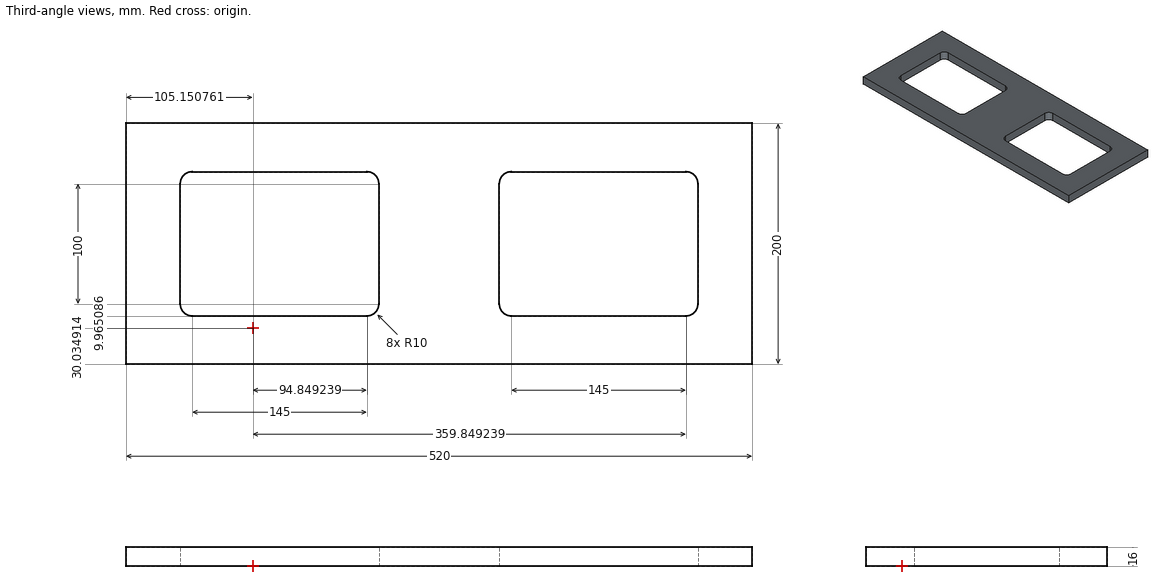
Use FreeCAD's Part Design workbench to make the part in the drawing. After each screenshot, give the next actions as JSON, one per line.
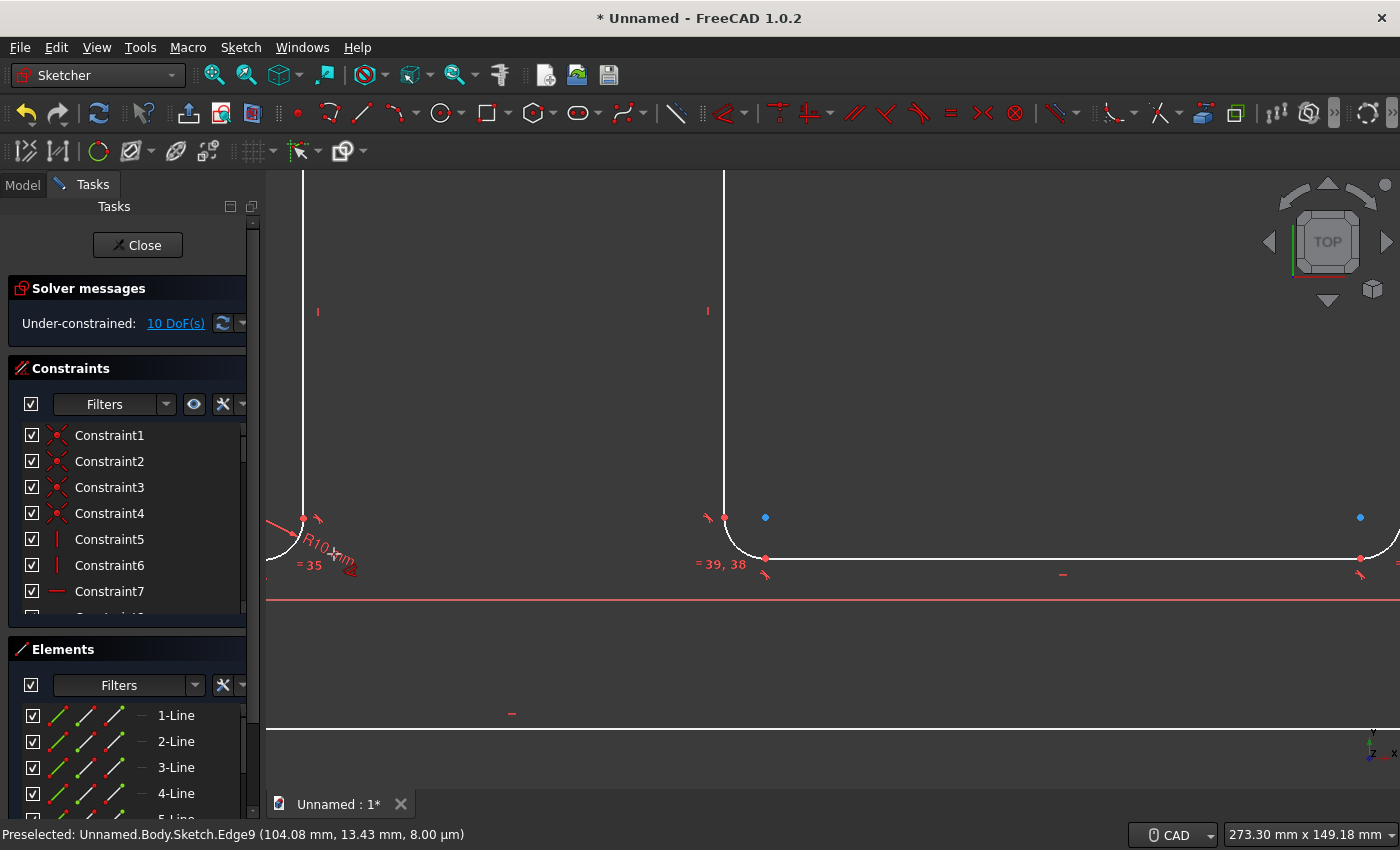
{"action": "left_click", "coordinate": [303, 228]}
{"action": "left_click", "coordinate": [337, 358]}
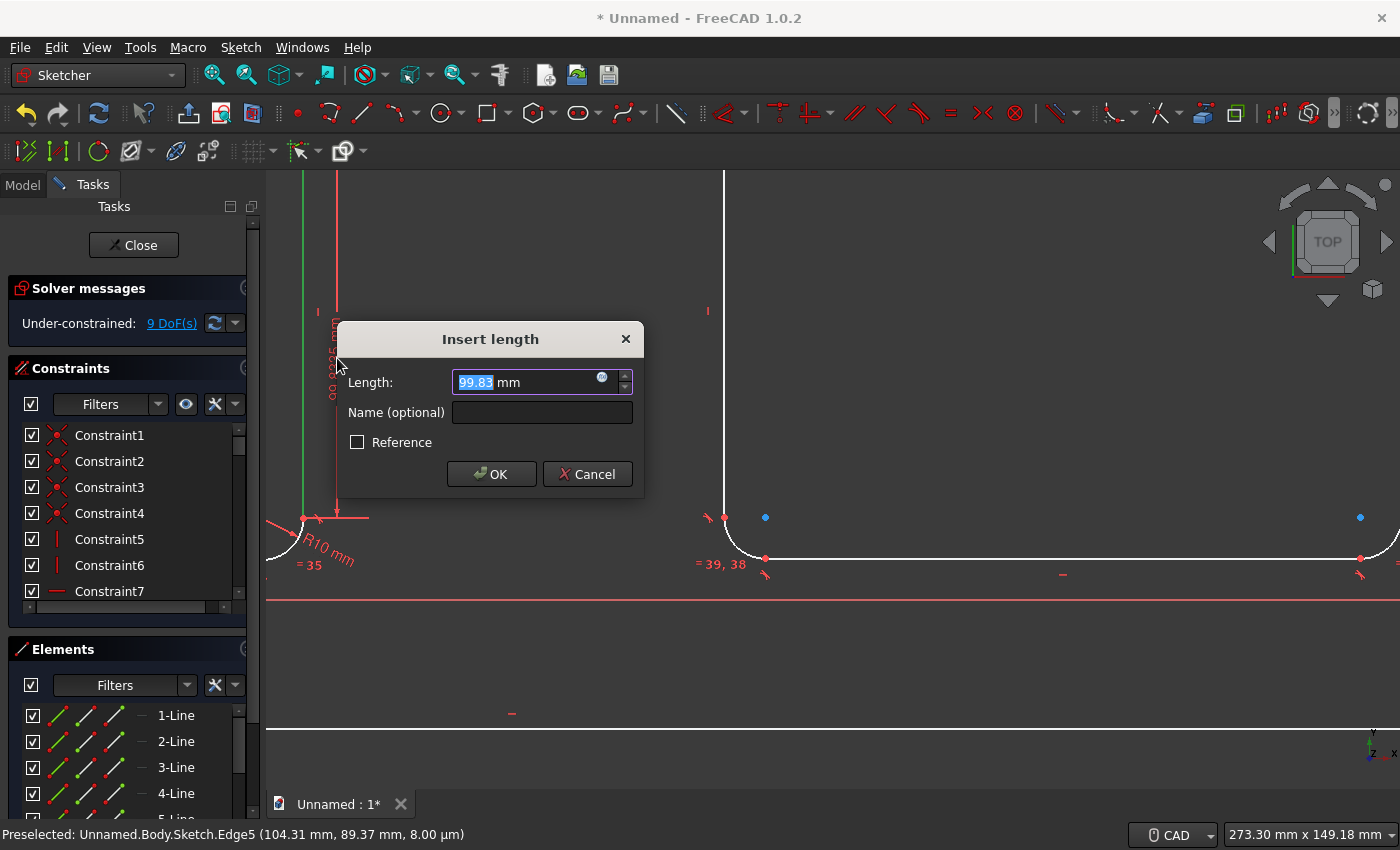
{"action": "type", "text": "100"}
{"action": "key", "text": "Return"}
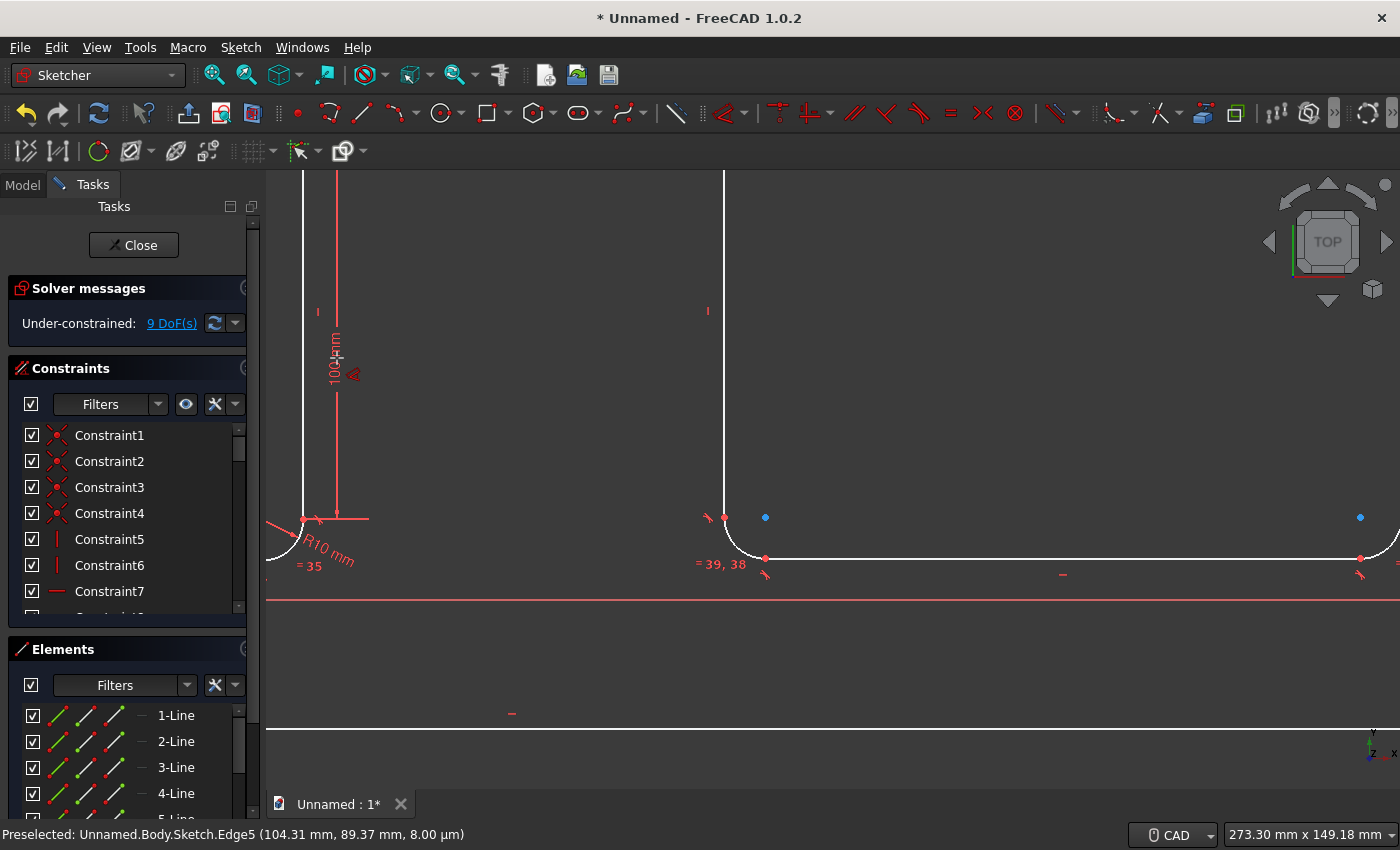
{"action": "scroll", "coordinate": [873, 553], "scroll_direction": "down", "scroll_amount": 6}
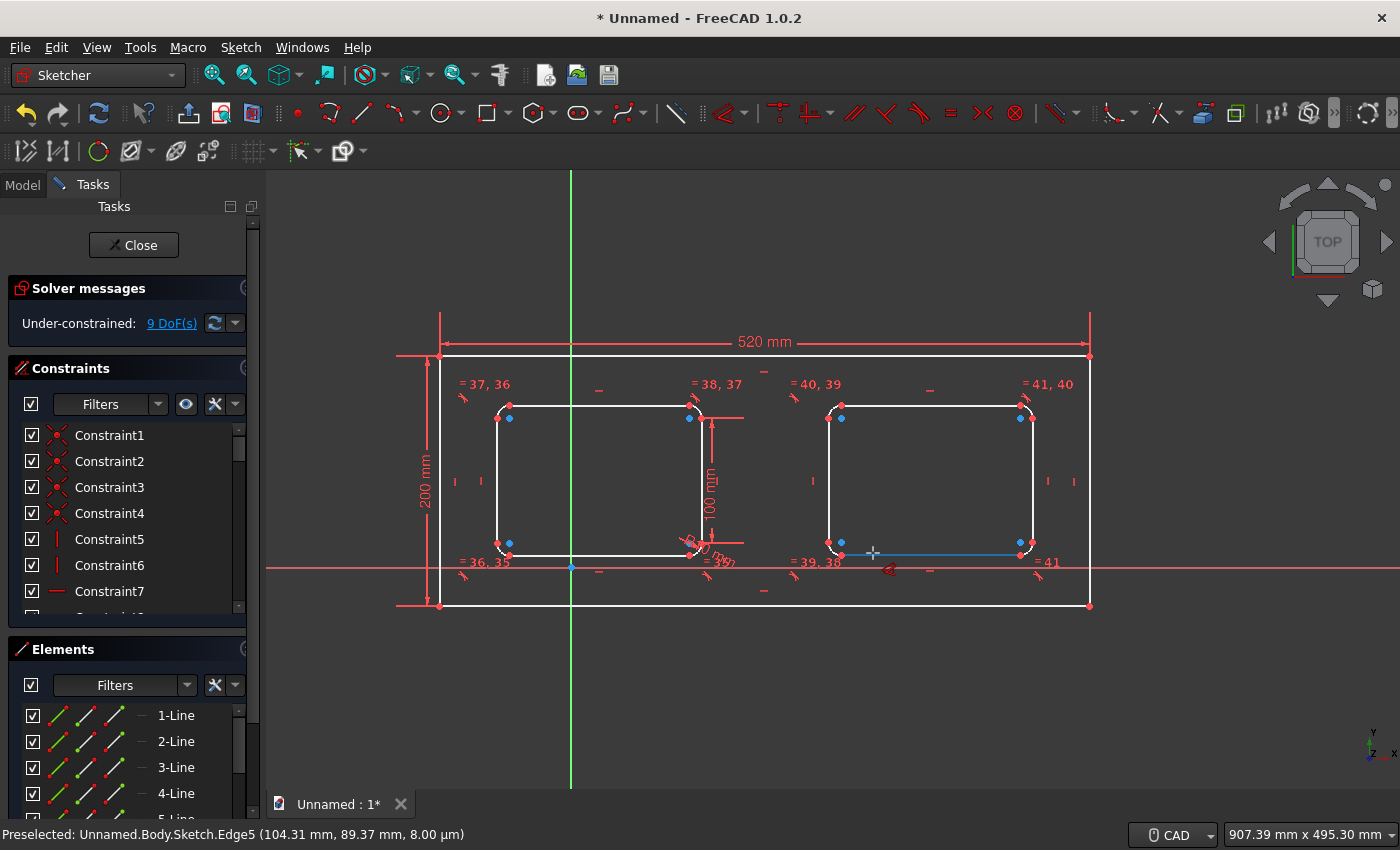
{"action": "left_click", "coordinate": [635, 556]}
{"action": "left_click", "coordinate": [599, 590]}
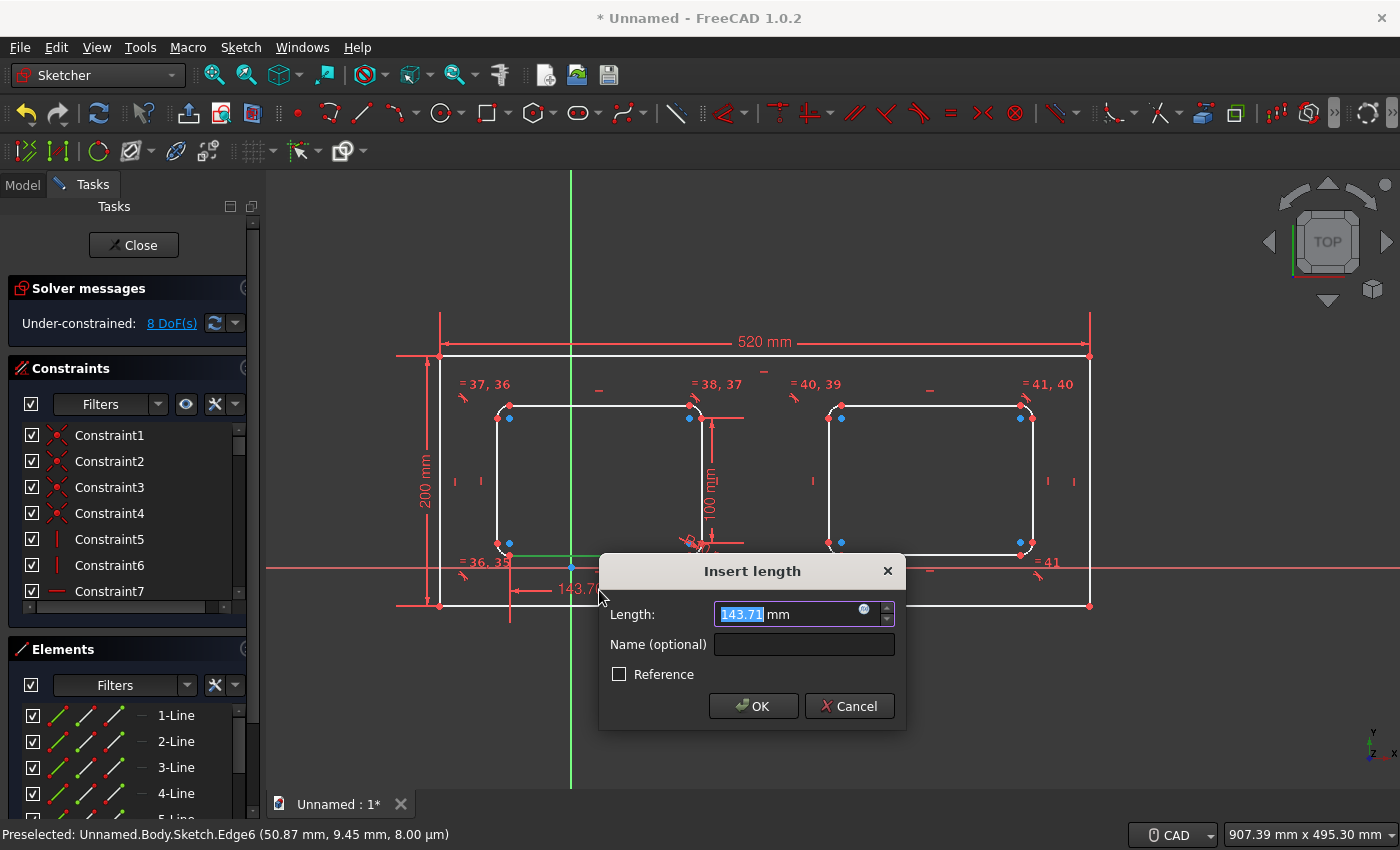
{"action": "type", "text": "145"}
{"action": "key", "text": "Return"}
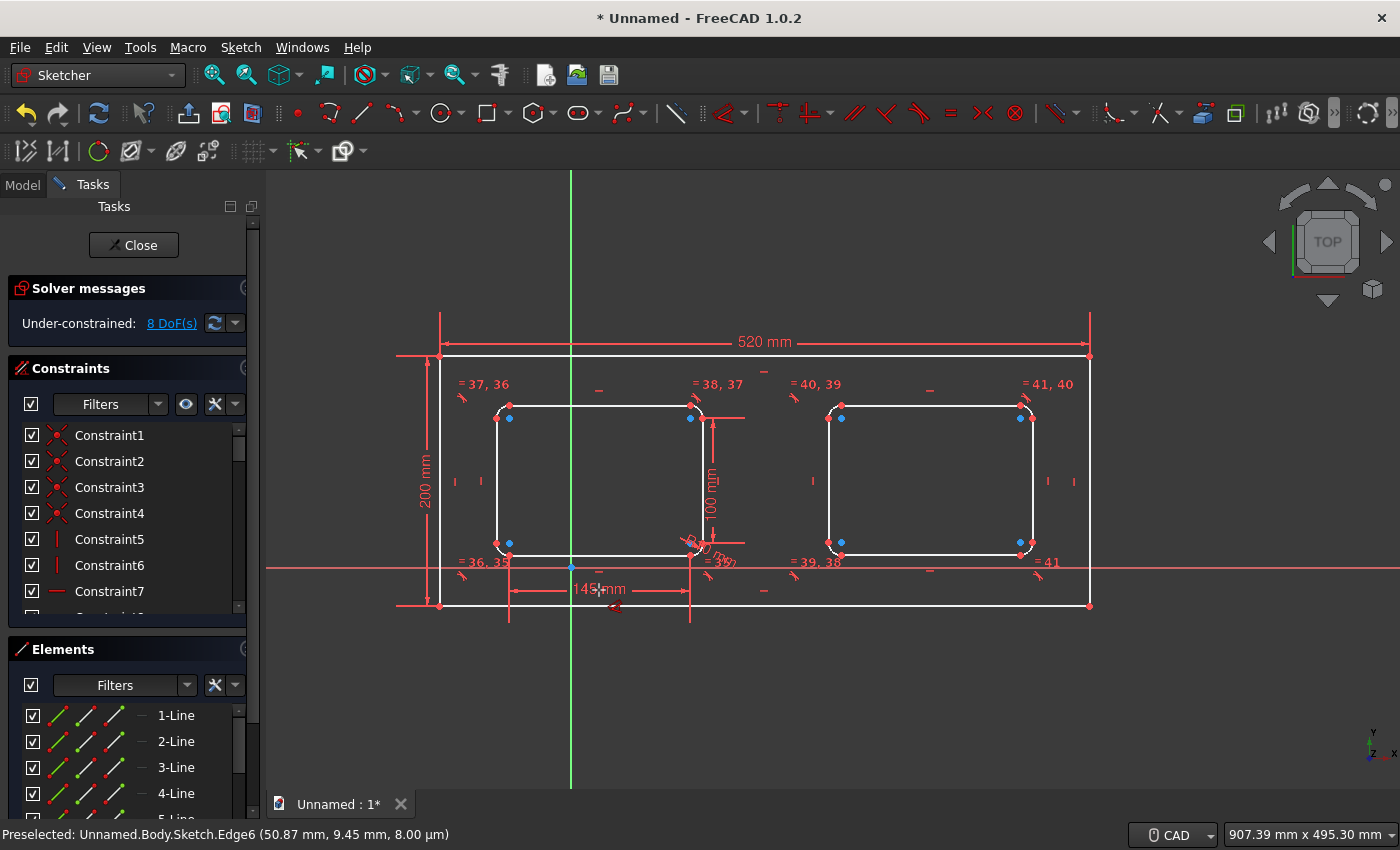
{"action": "left_click", "coordinate": [966, 555]}
{"action": "left_click", "coordinate": [931, 589]}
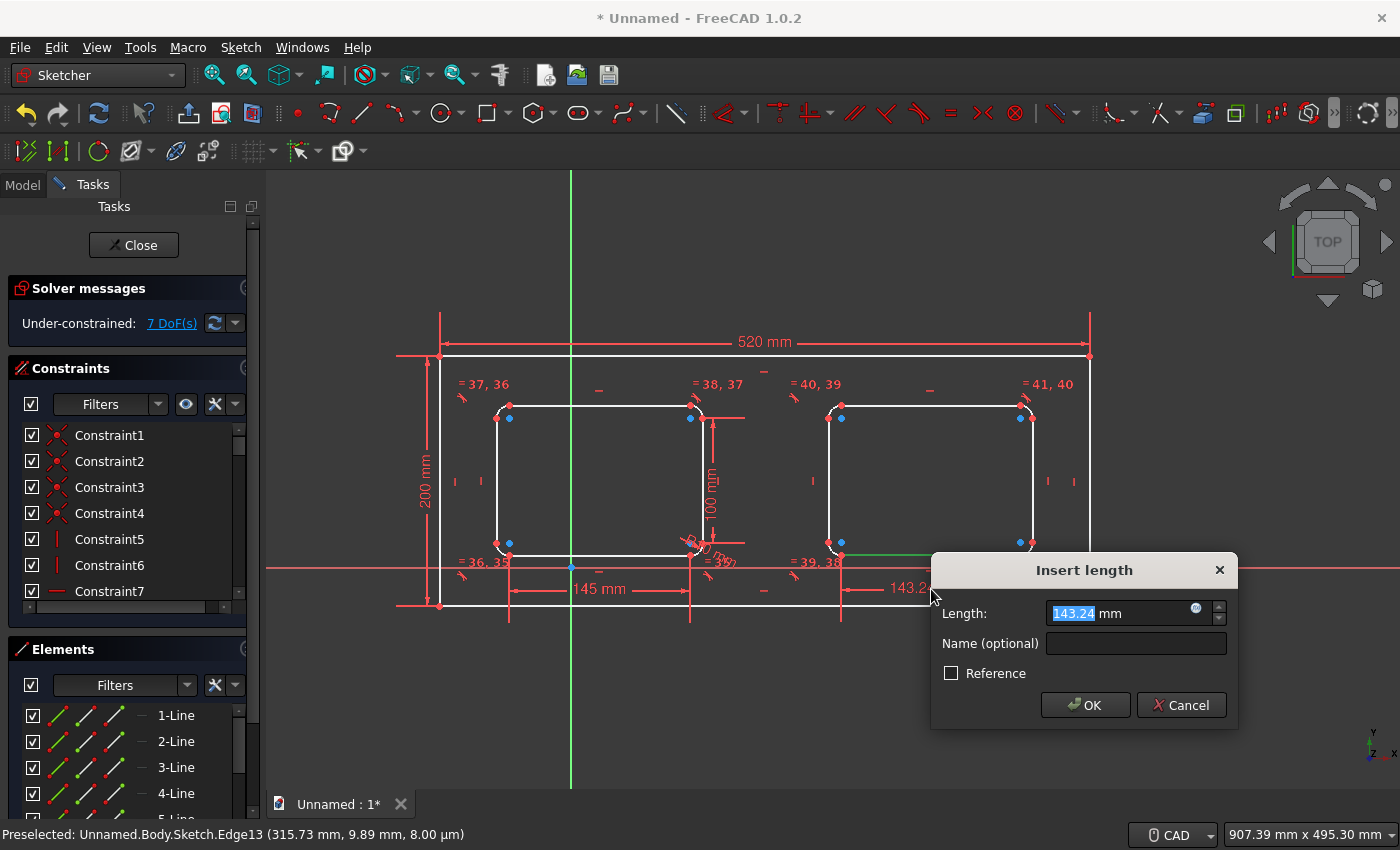
{"action": "type", "text": "145"}
{"action": "key", "text": "Return"}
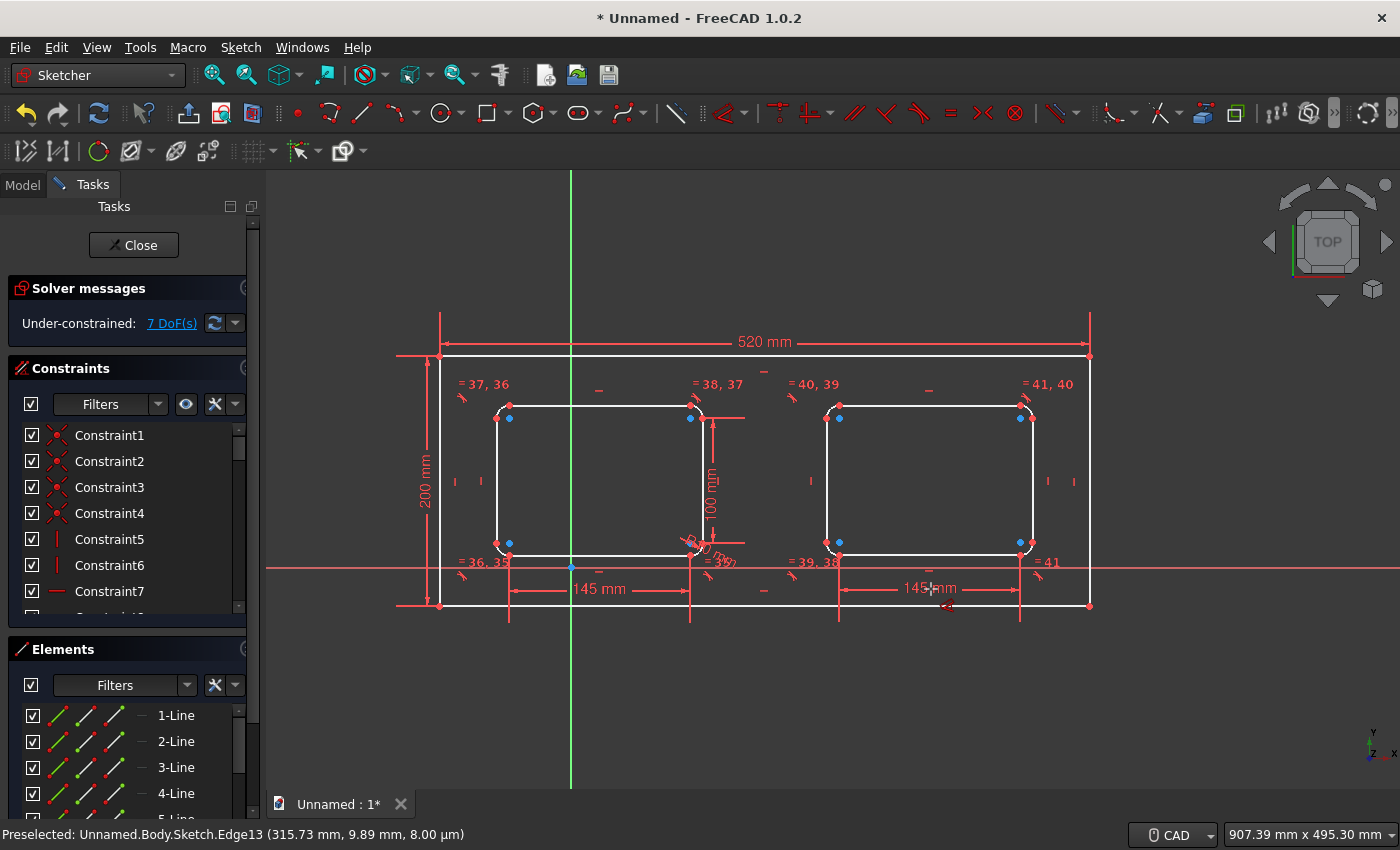
{"action": "left_click", "coordinate": [827, 505]}
{"action": "left_click", "coordinate": [861, 480]}